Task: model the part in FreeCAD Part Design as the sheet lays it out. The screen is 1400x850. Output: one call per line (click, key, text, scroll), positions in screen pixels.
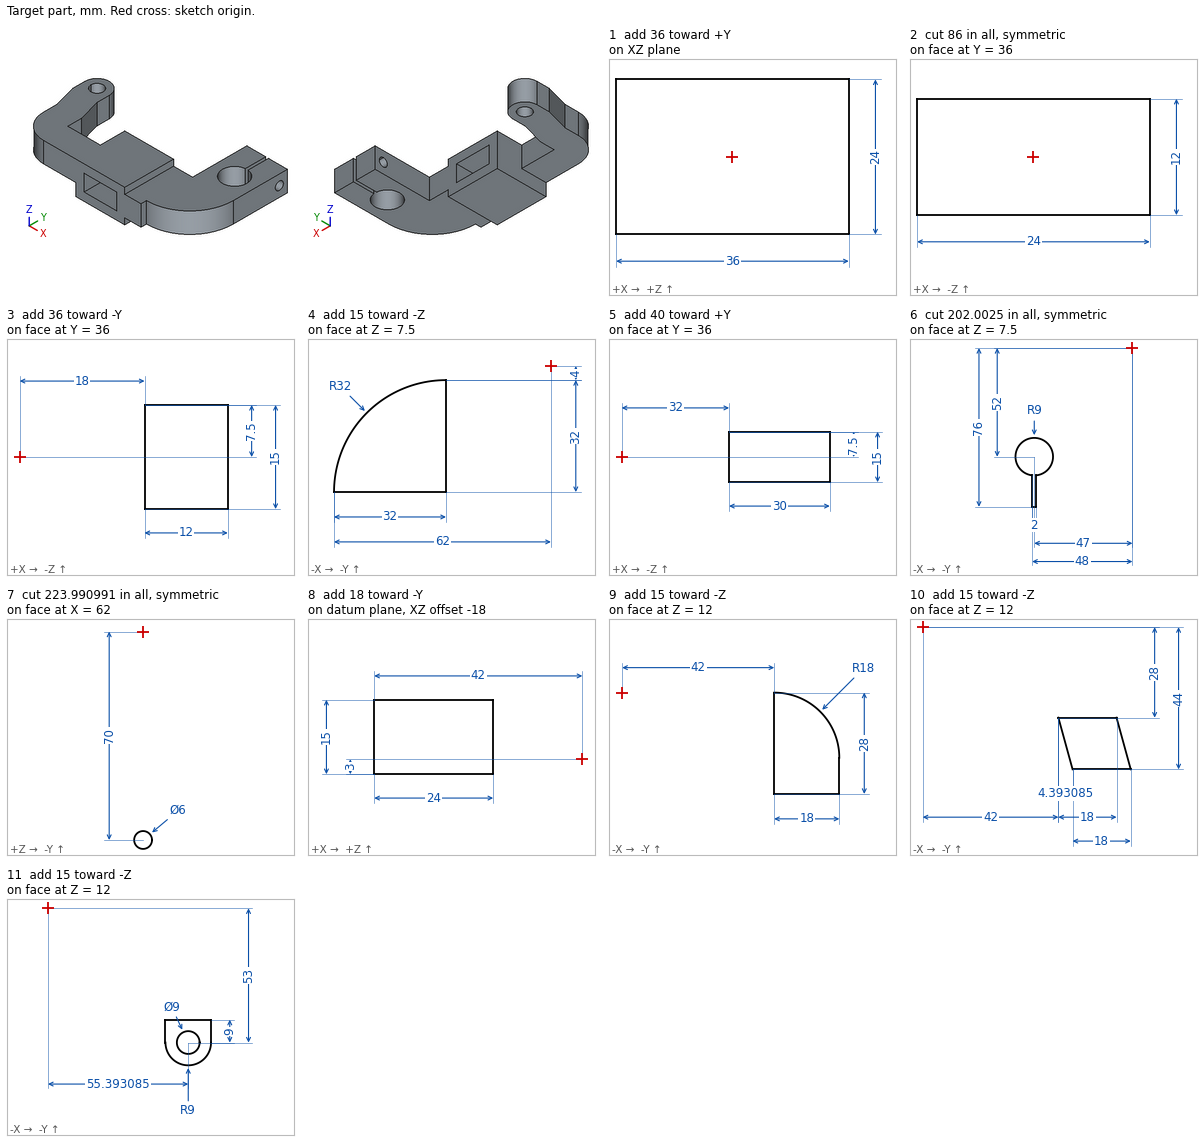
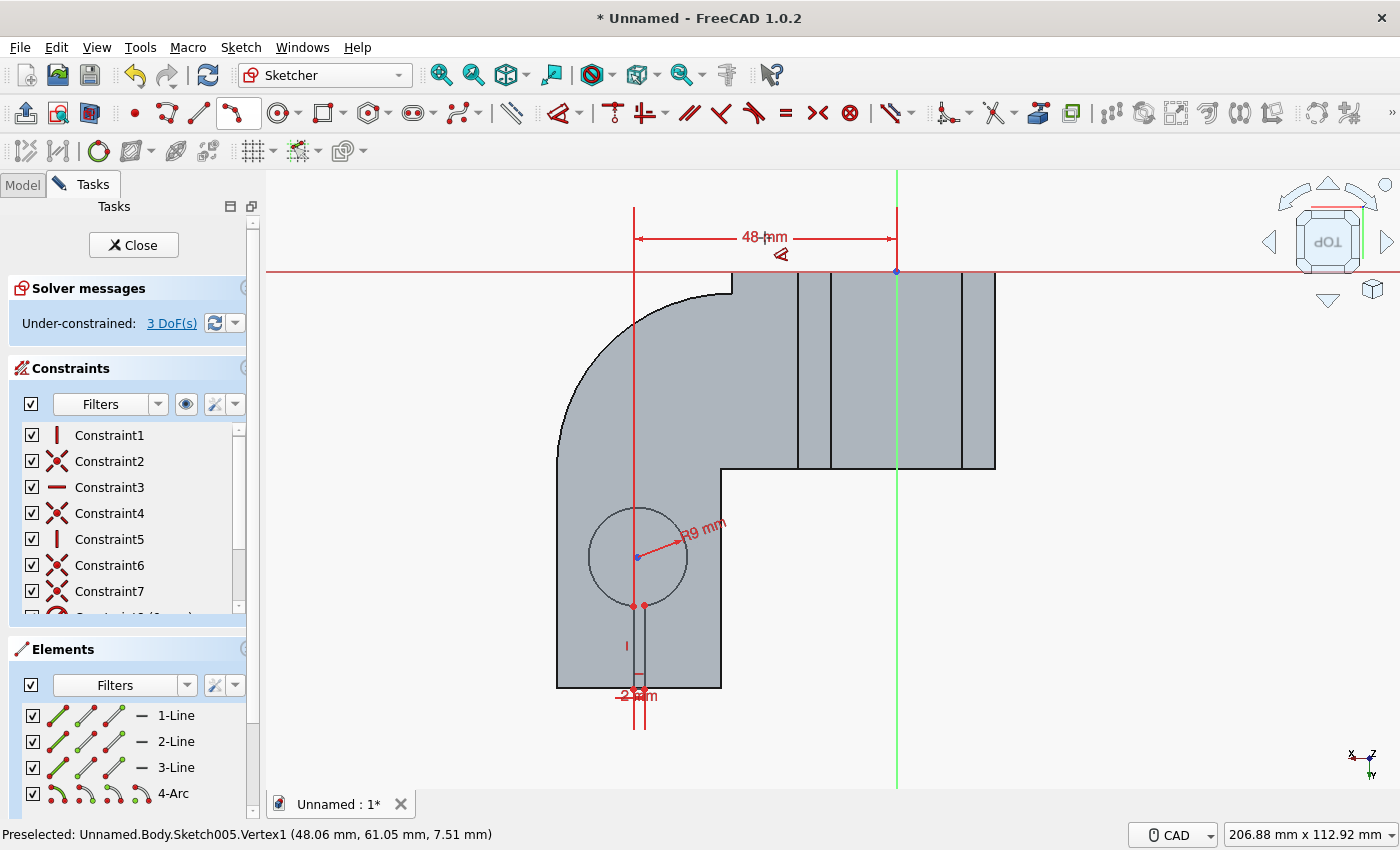
click(634, 689)
click(931, 480)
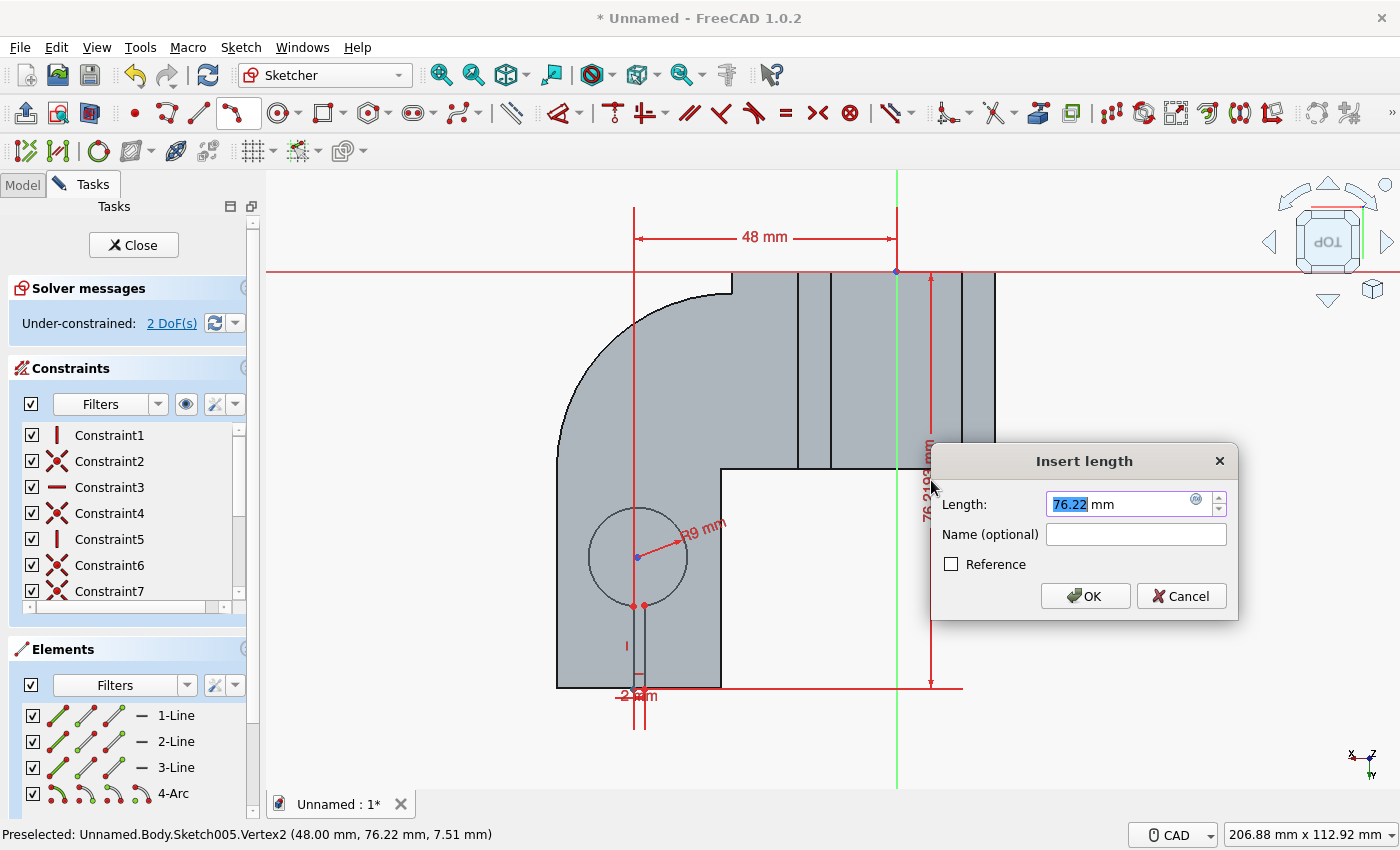
text(76)
key(Return)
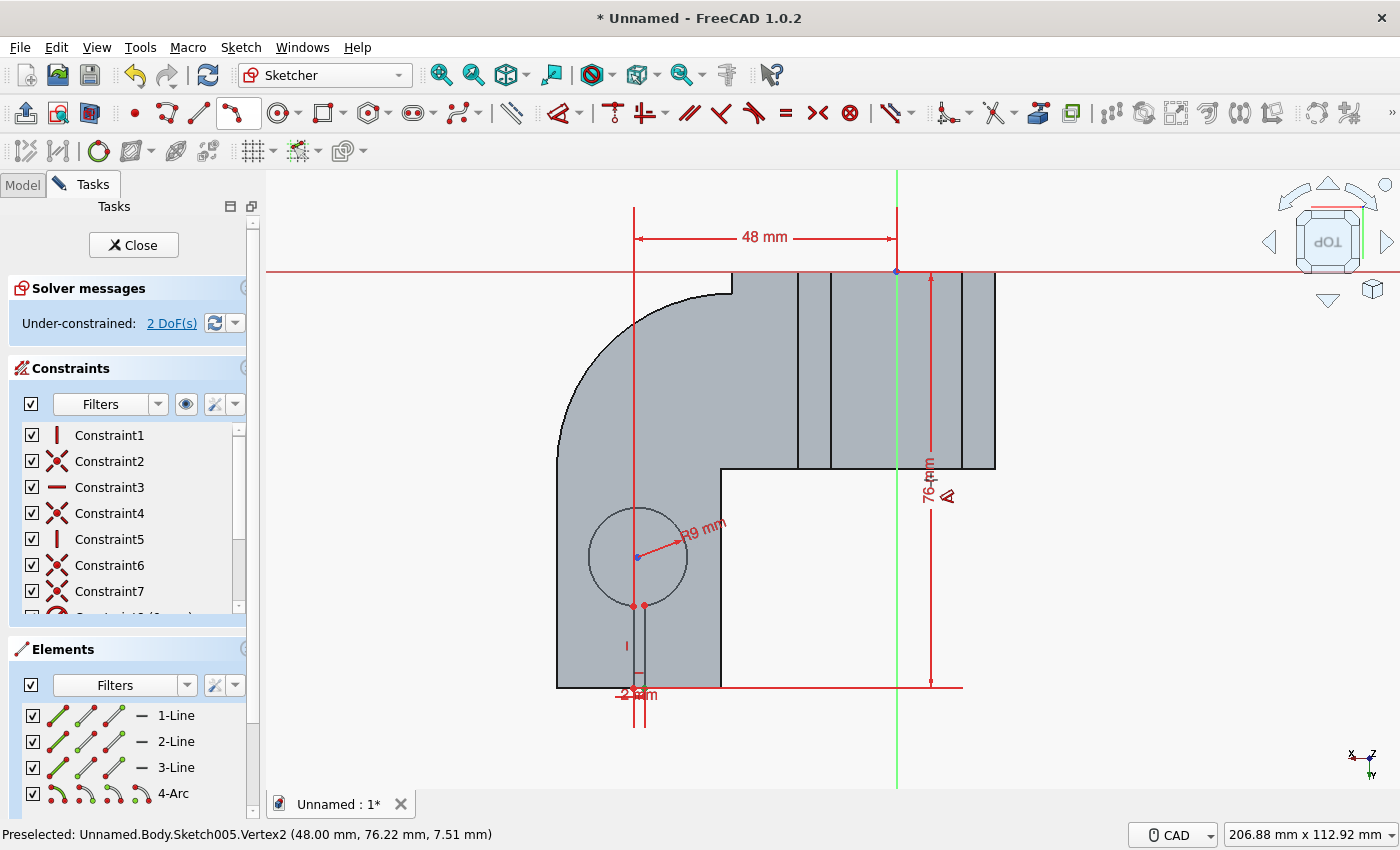
click(638, 557)
click(677, 238)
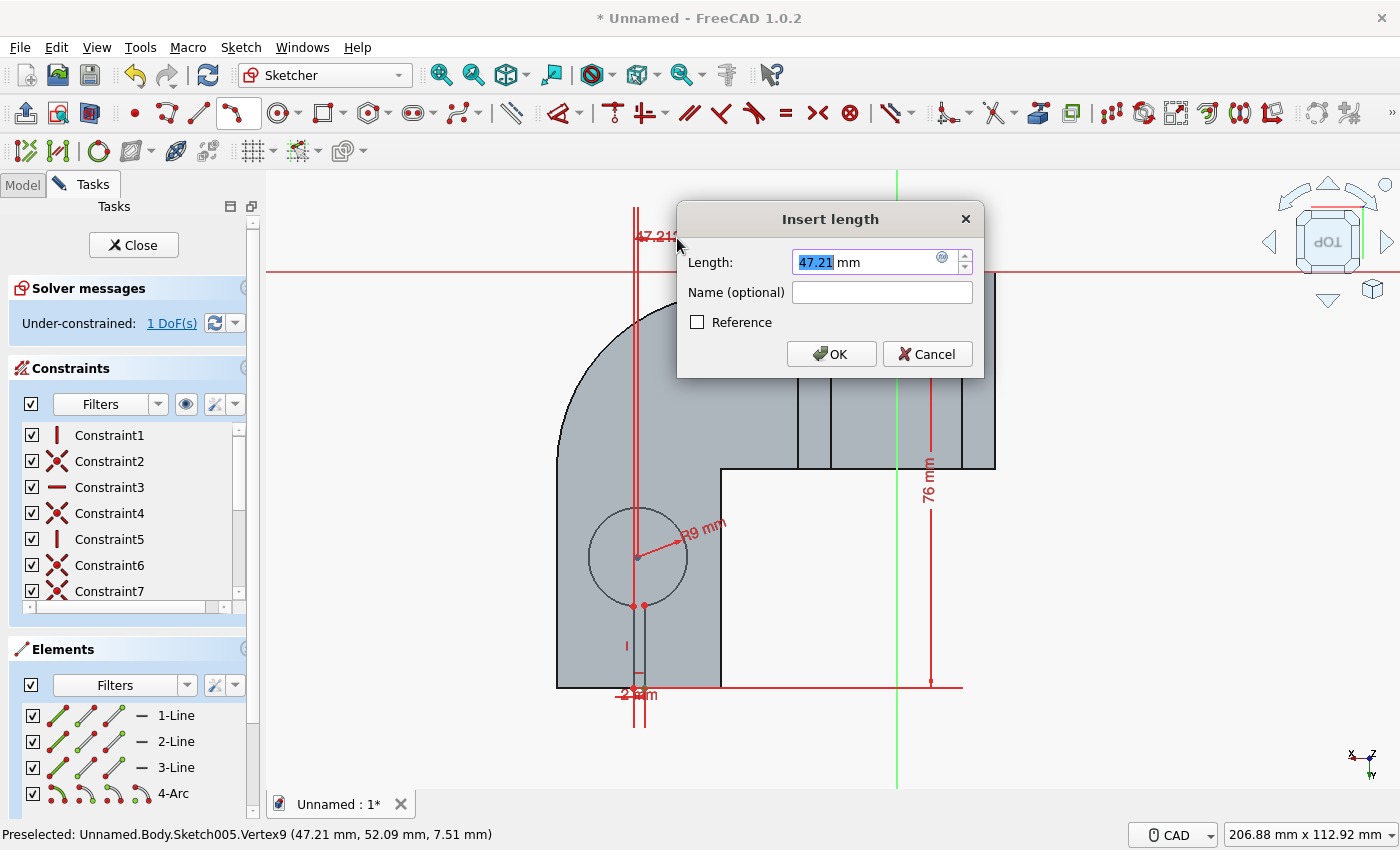
text(47)
key(Return)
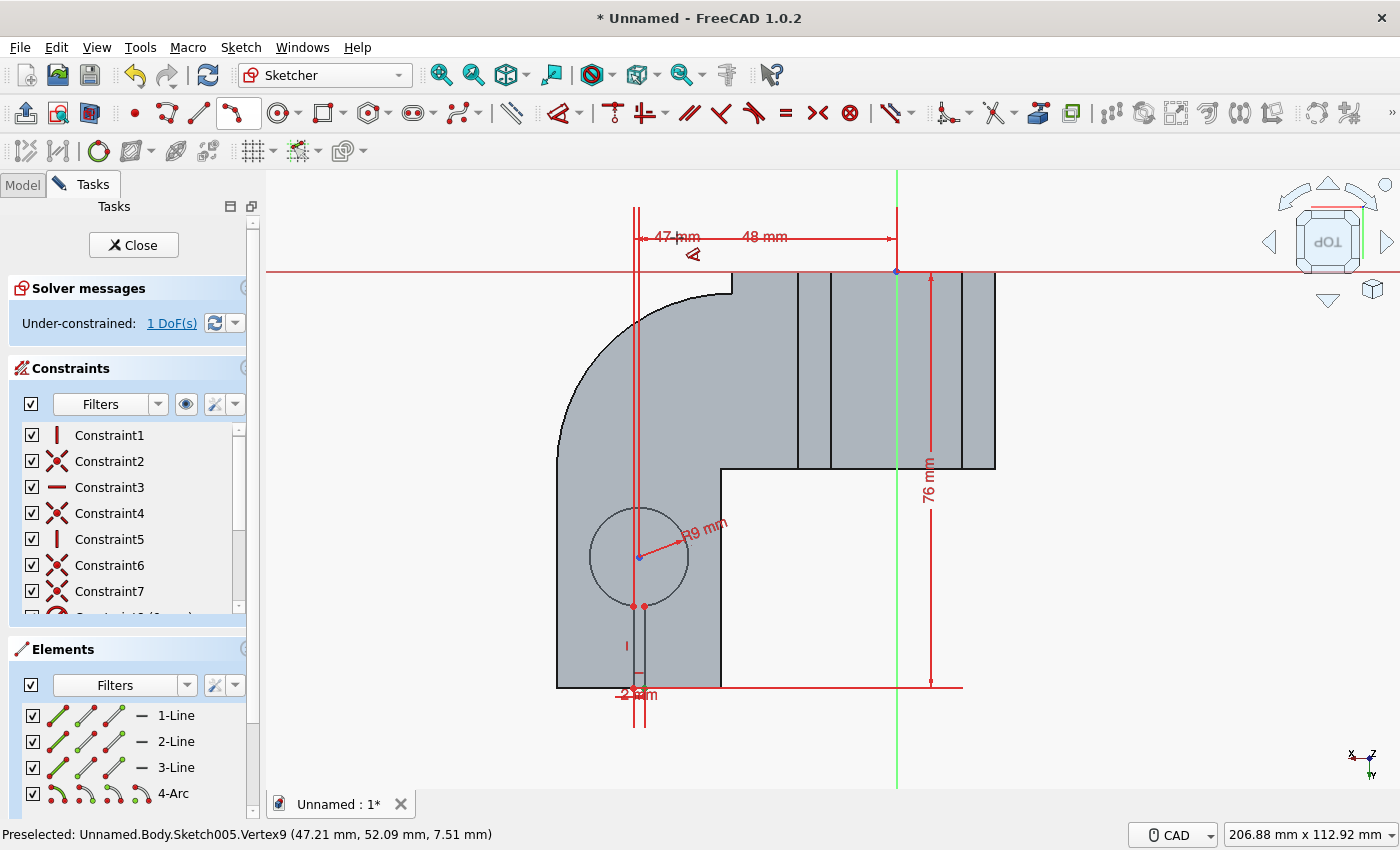
click(639, 557)
click(931, 414)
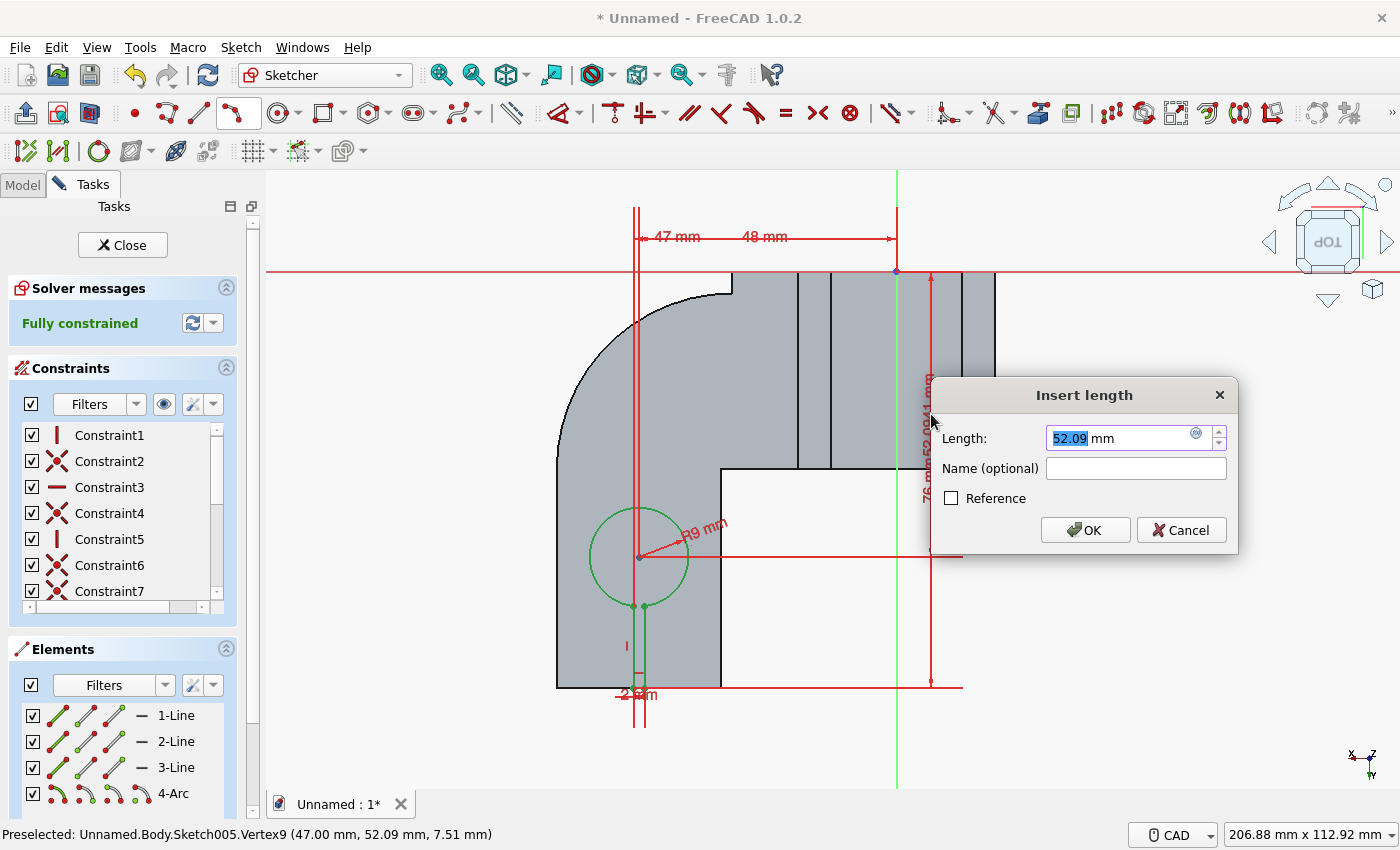
text(52)
key(Return)
key(Escape)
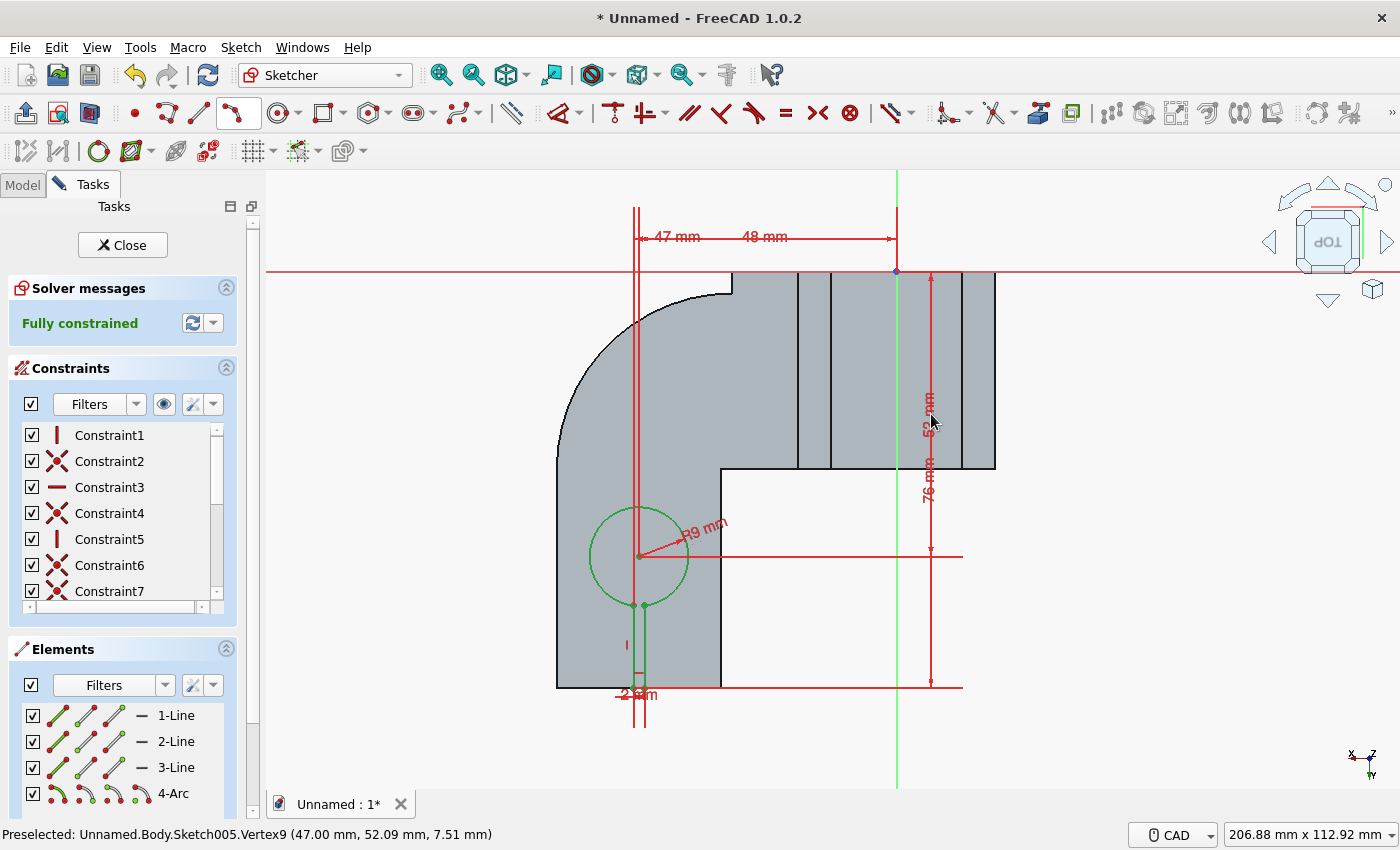
click(123, 245)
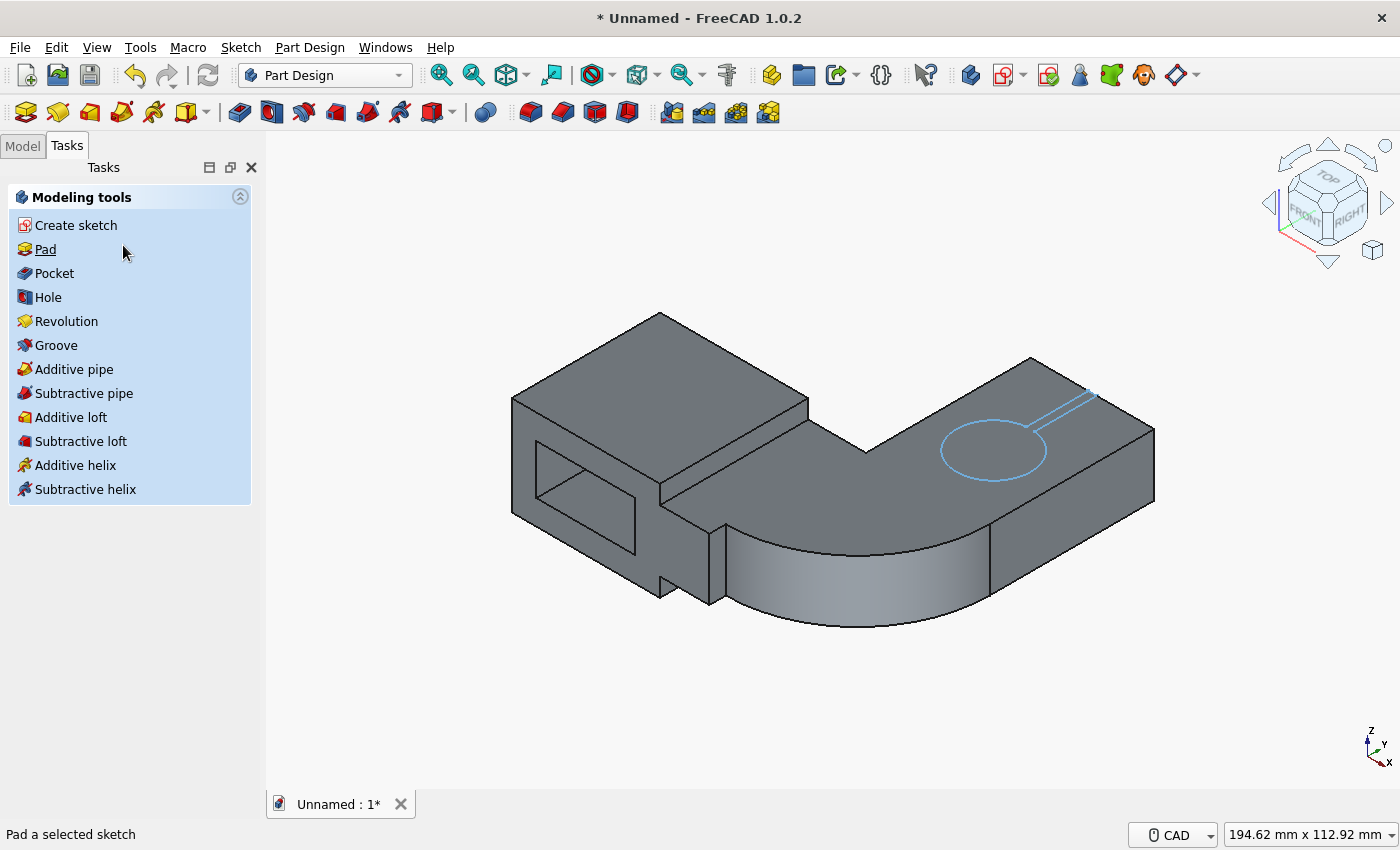
click(240, 112)